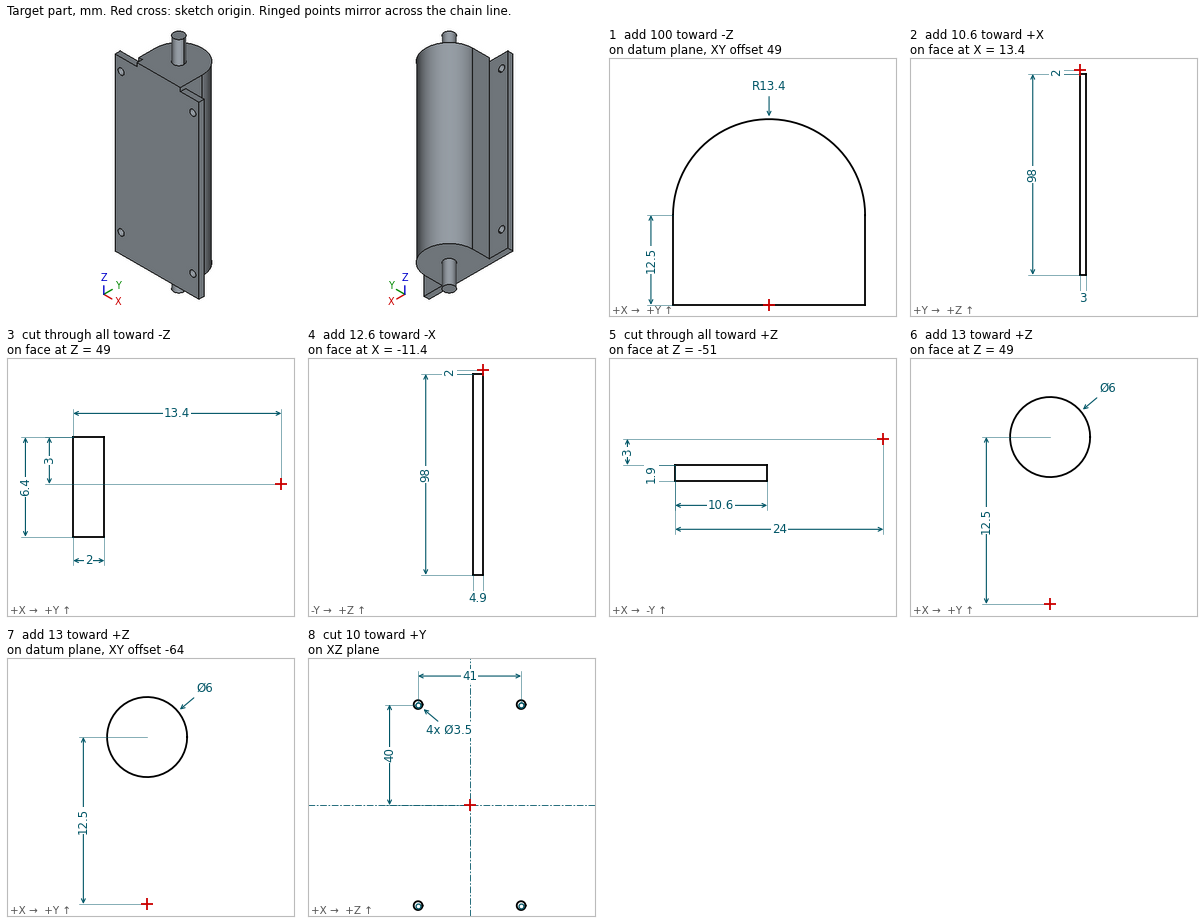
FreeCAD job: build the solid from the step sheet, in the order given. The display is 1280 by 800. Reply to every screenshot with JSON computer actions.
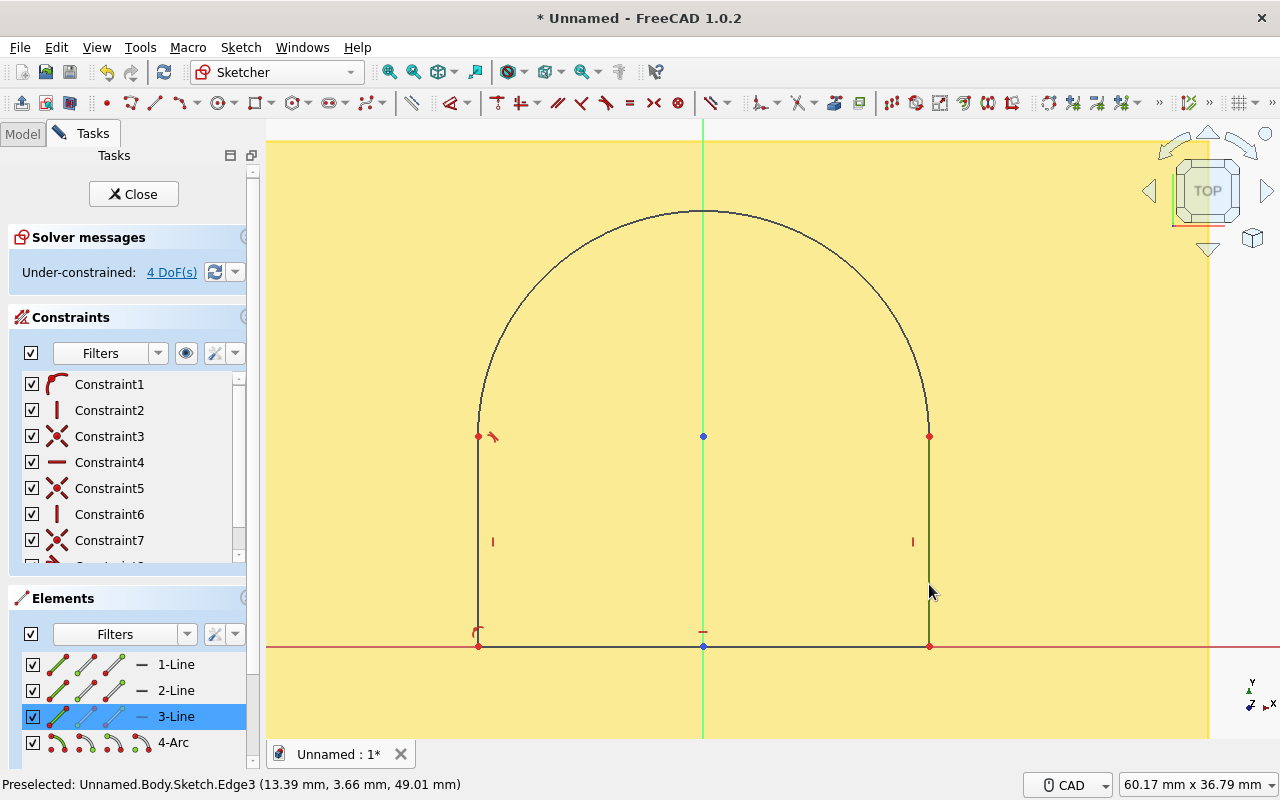
{"action": "left_click", "coordinate": [836, 254]}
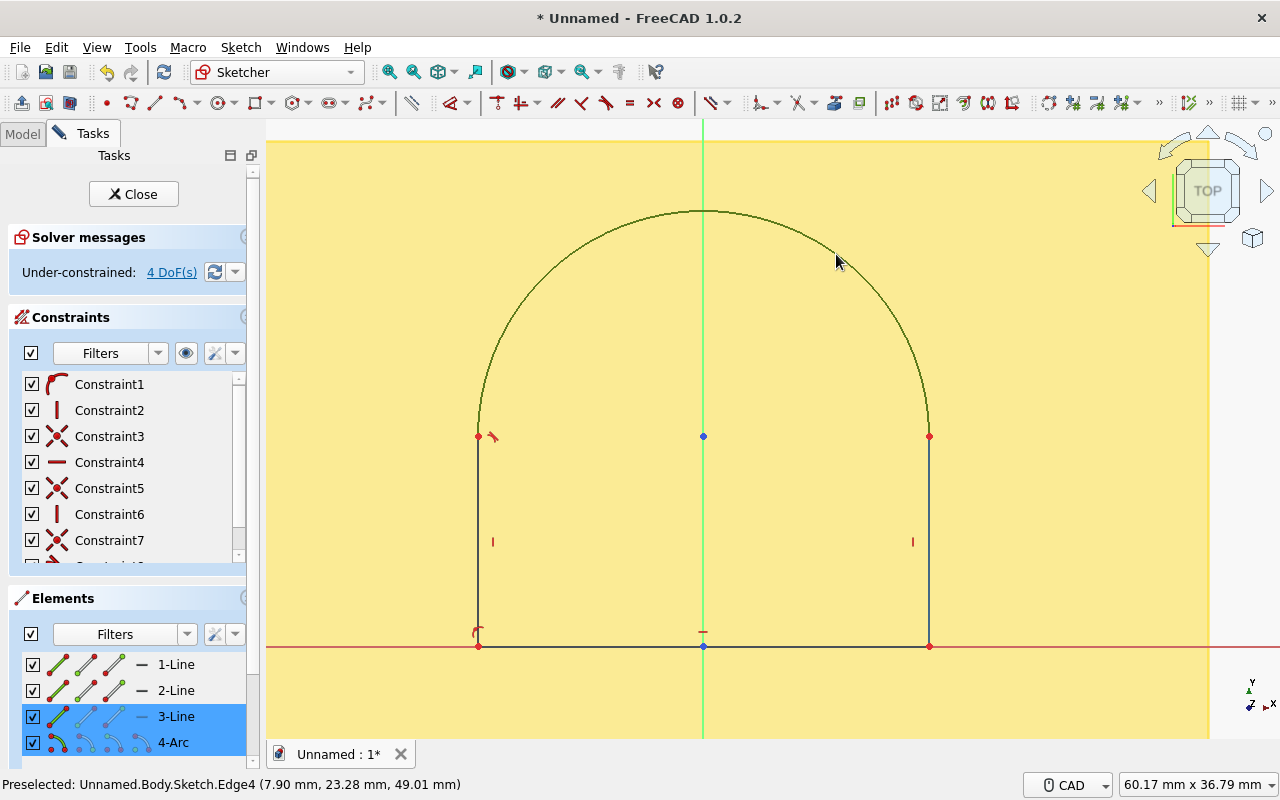
{"action": "left_click", "coordinate": [606, 104]}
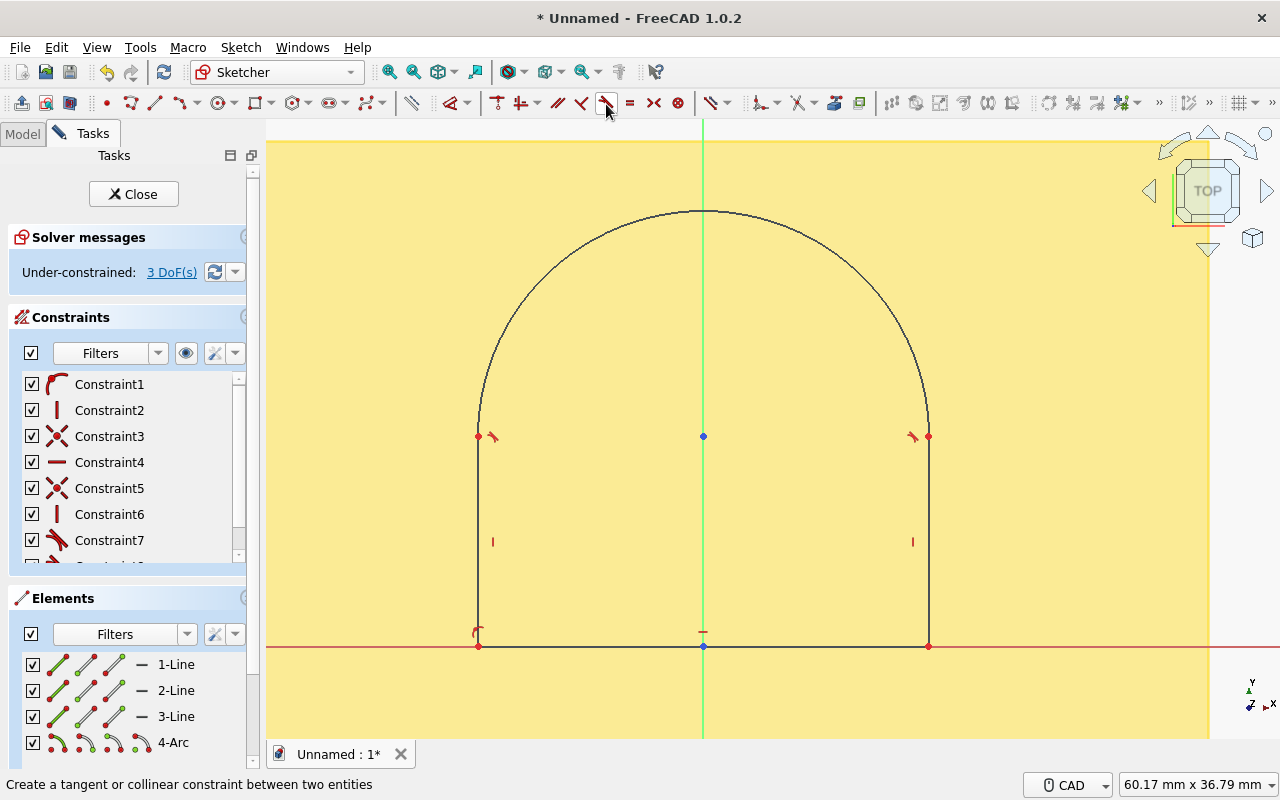
{"action": "left_click", "coordinate": [703, 437]}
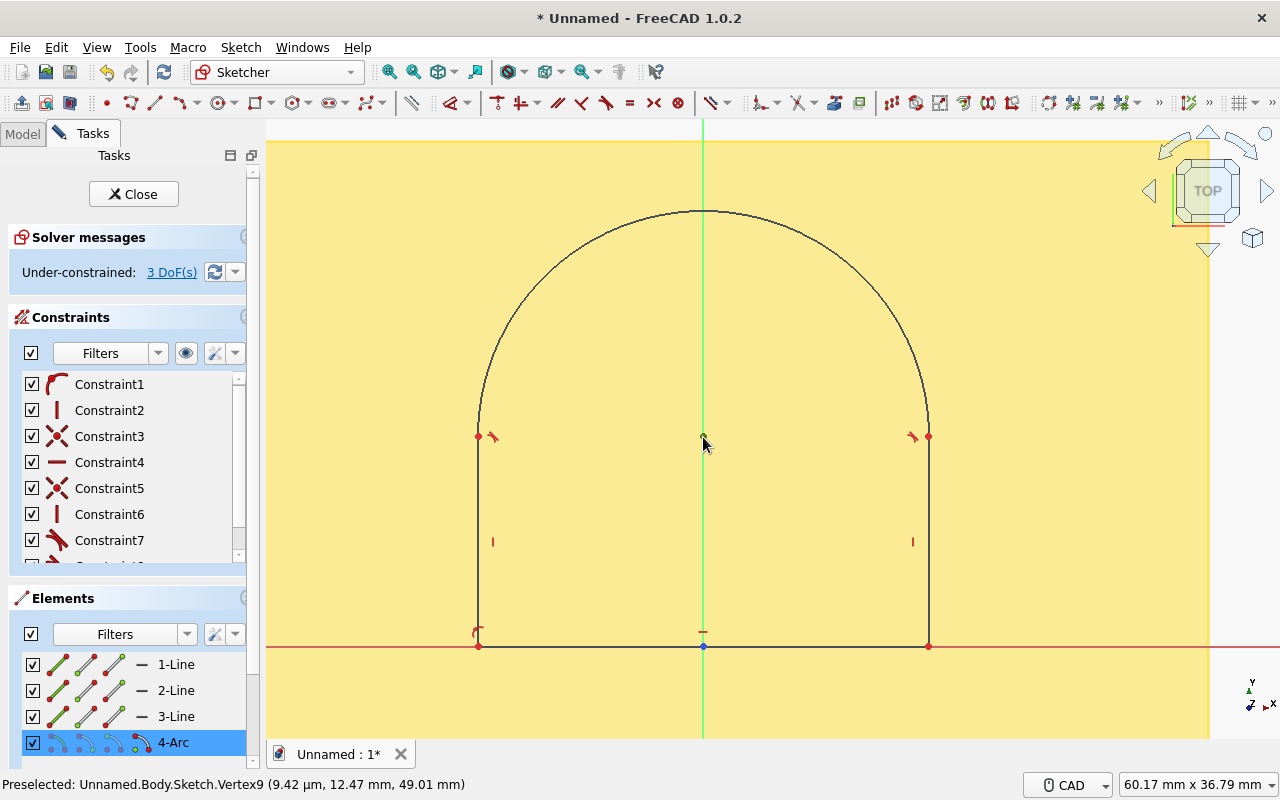
{"action": "left_click", "coordinate": [703, 590]}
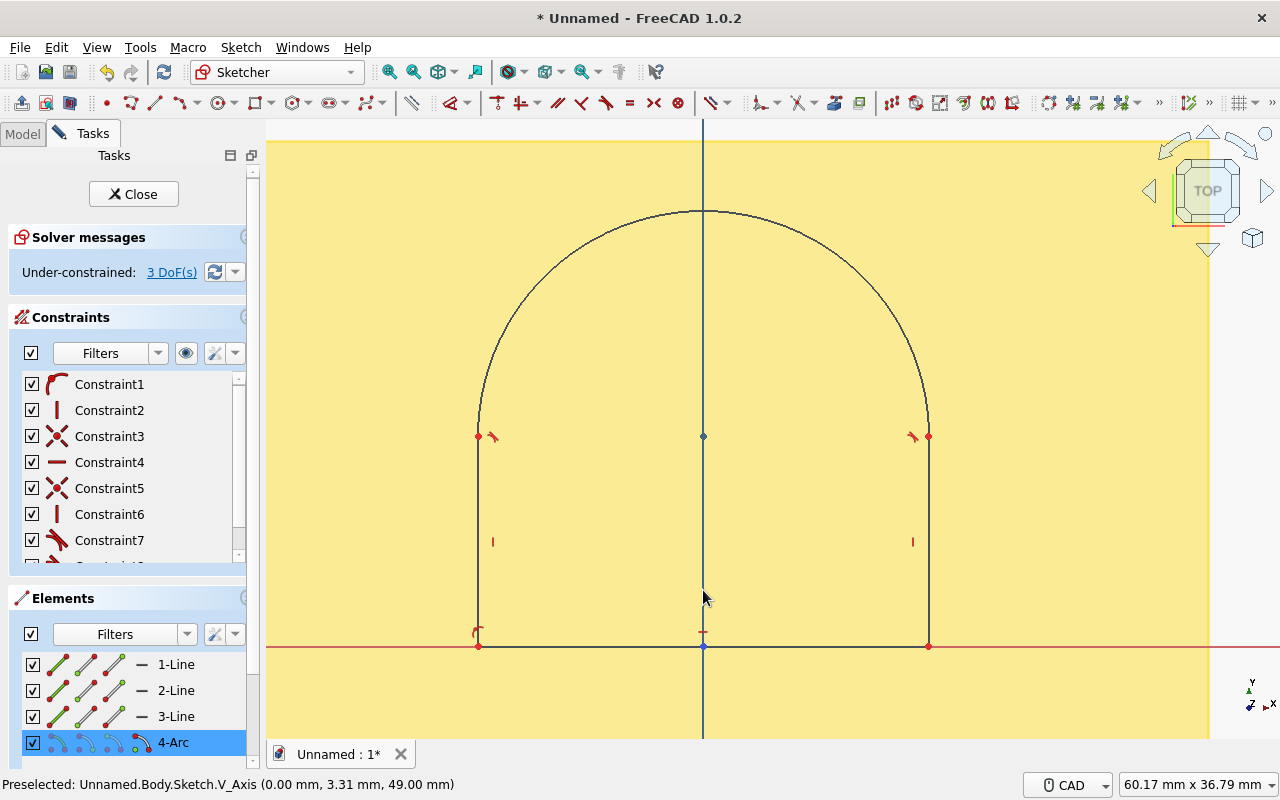
{"action": "left_click", "coordinate": [498, 104]}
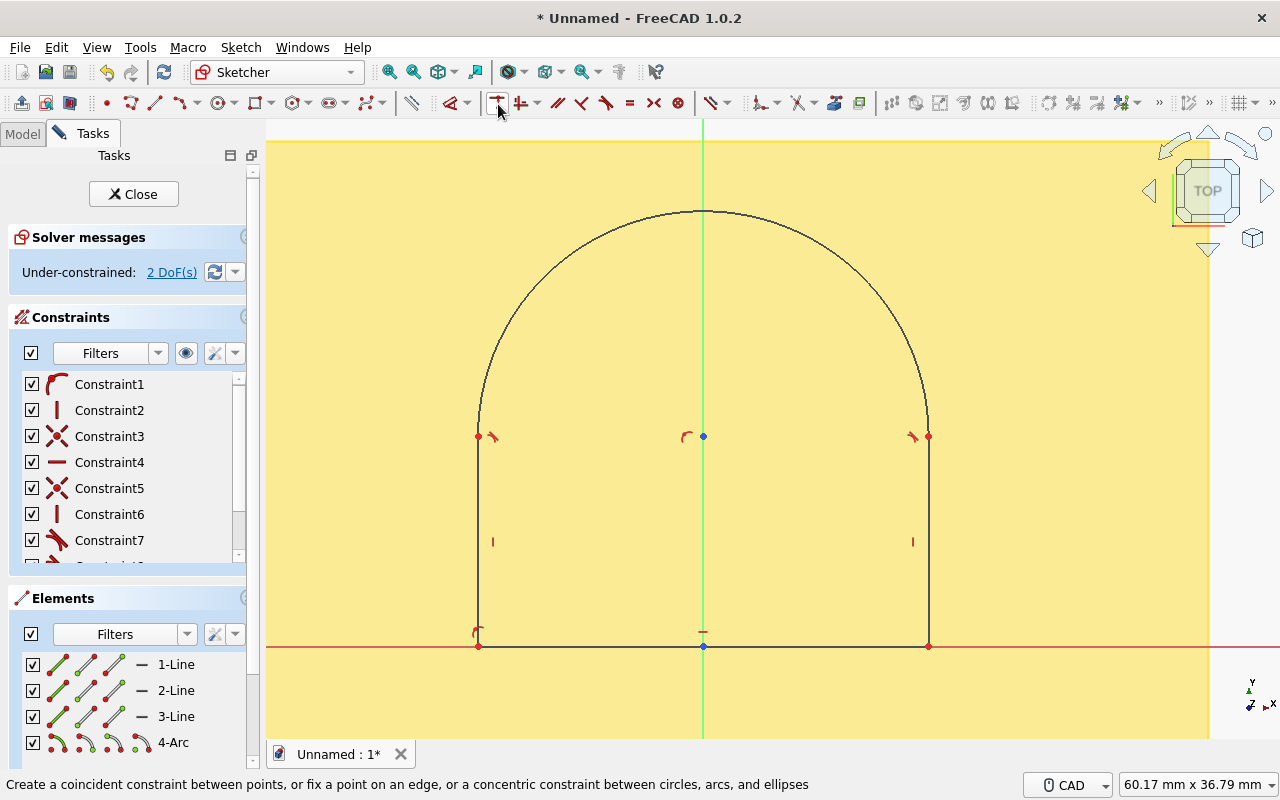
{"action": "left_click", "coordinate": [450, 104]}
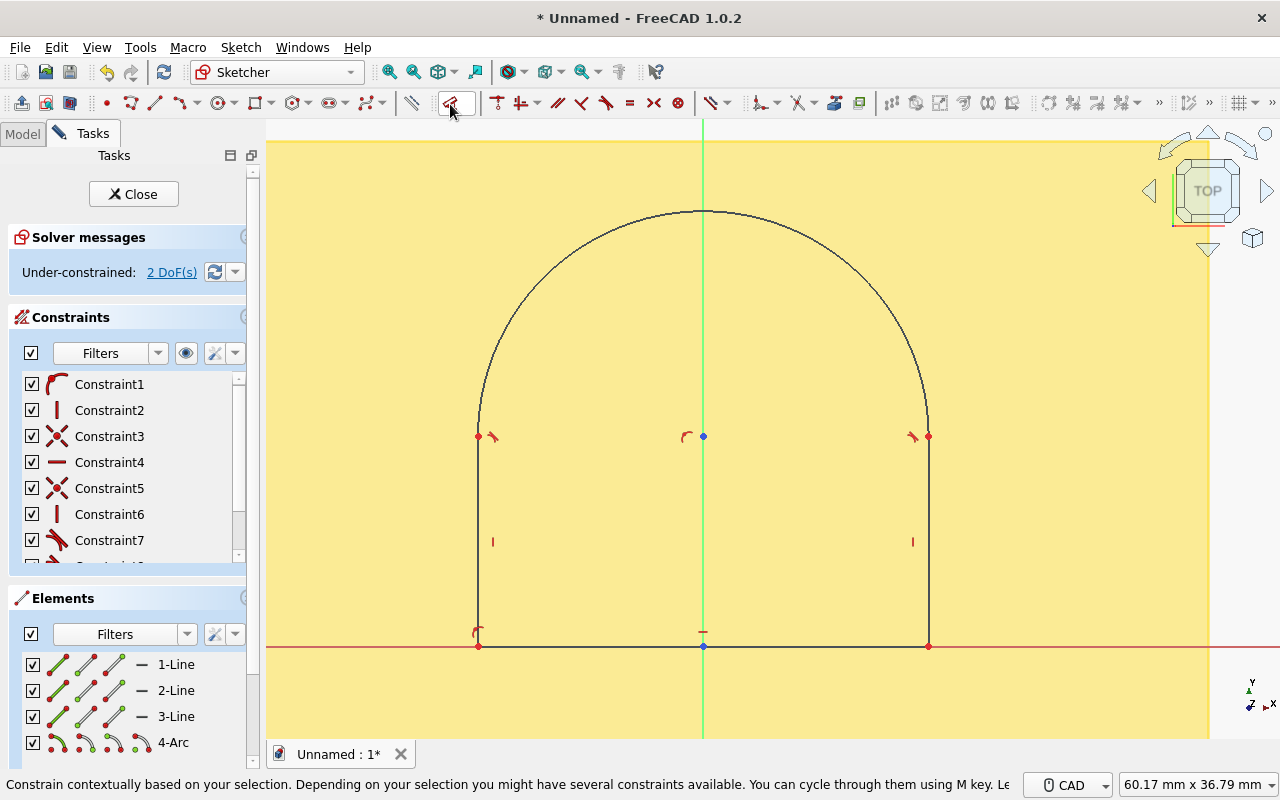
{"action": "left_click", "coordinate": [836, 254]}
{"action": "left_click", "coordinate": [855, 228]}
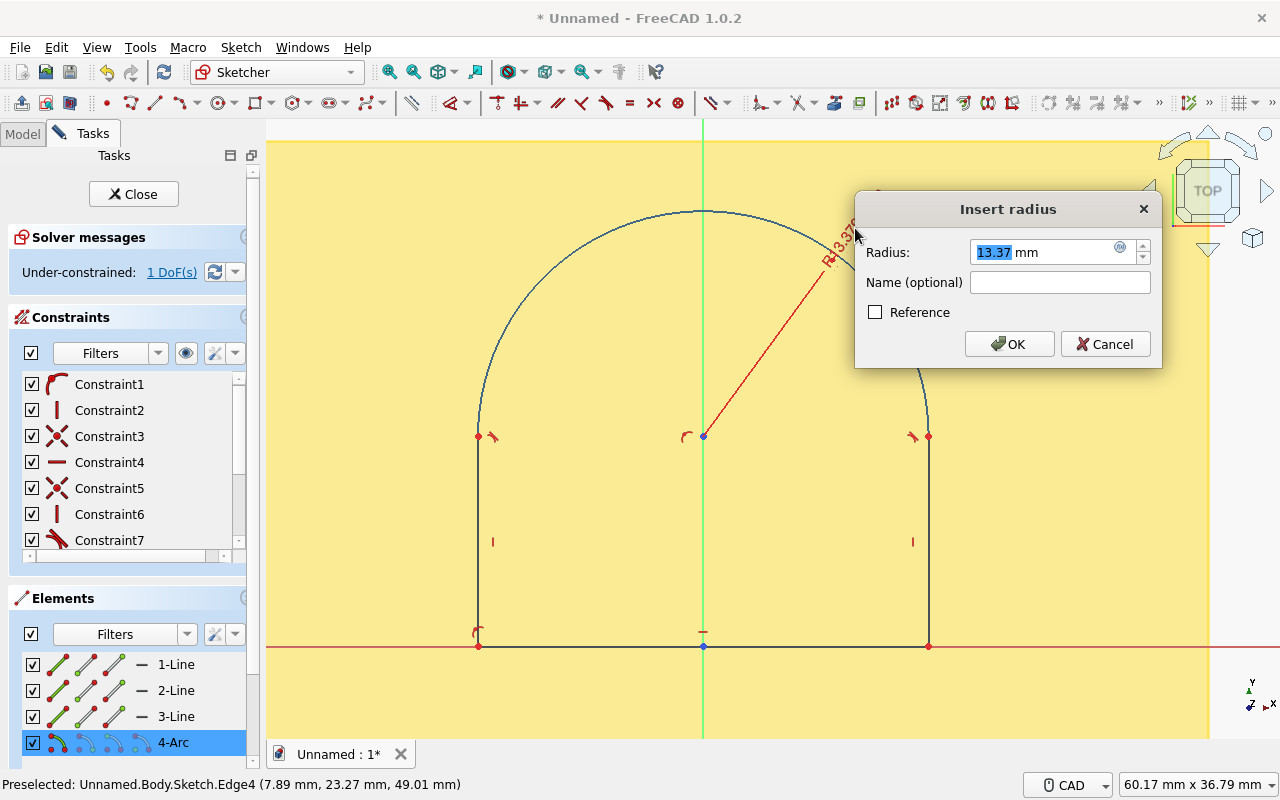
{"action": "type", "text": "13.4"}
{"action": "key", "text": "Return"}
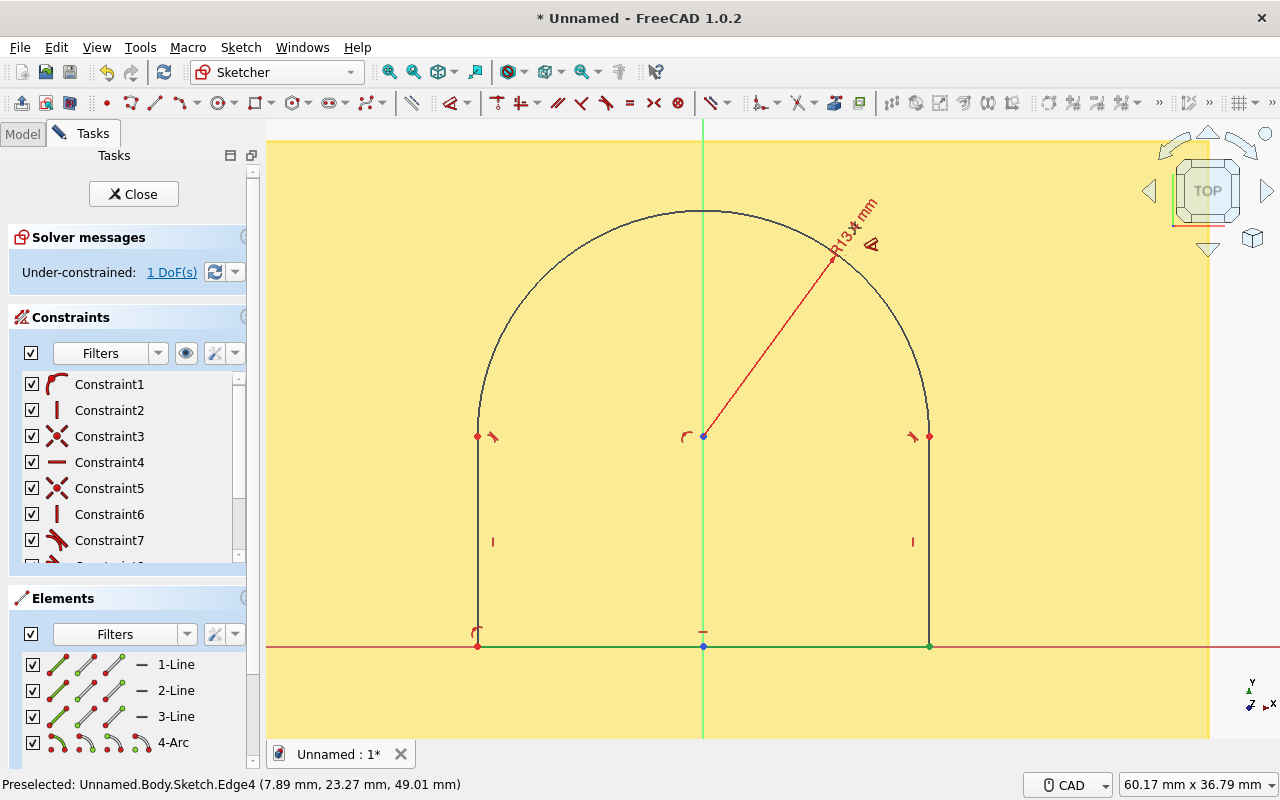
{"action": "left_click", "coordinate": [478, 500]}
{"action": "left_click", "coordinate": [444, 542]}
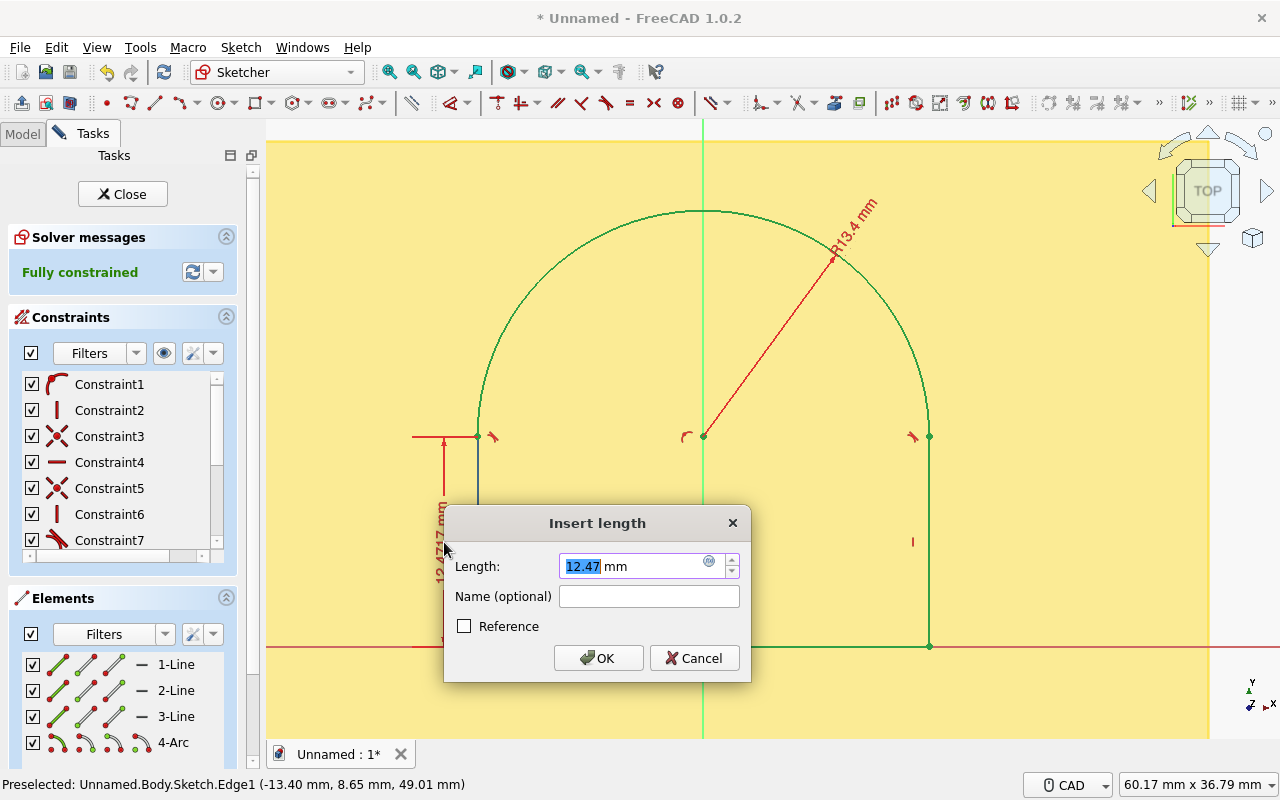
{"action": "type", "text": "12.5"}
{"action": "key", "text": "Return"}
{"action": "key", "text": "Escape"}